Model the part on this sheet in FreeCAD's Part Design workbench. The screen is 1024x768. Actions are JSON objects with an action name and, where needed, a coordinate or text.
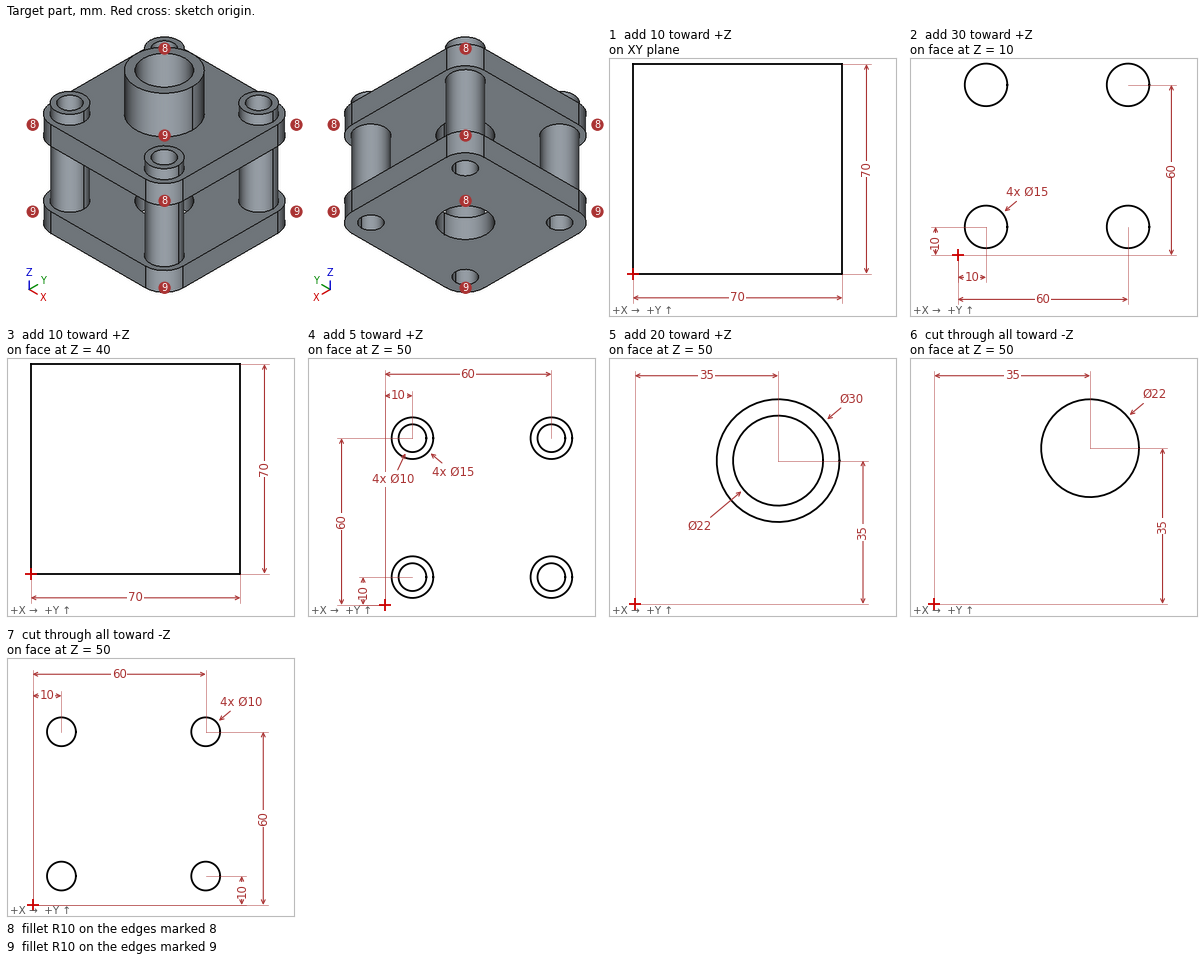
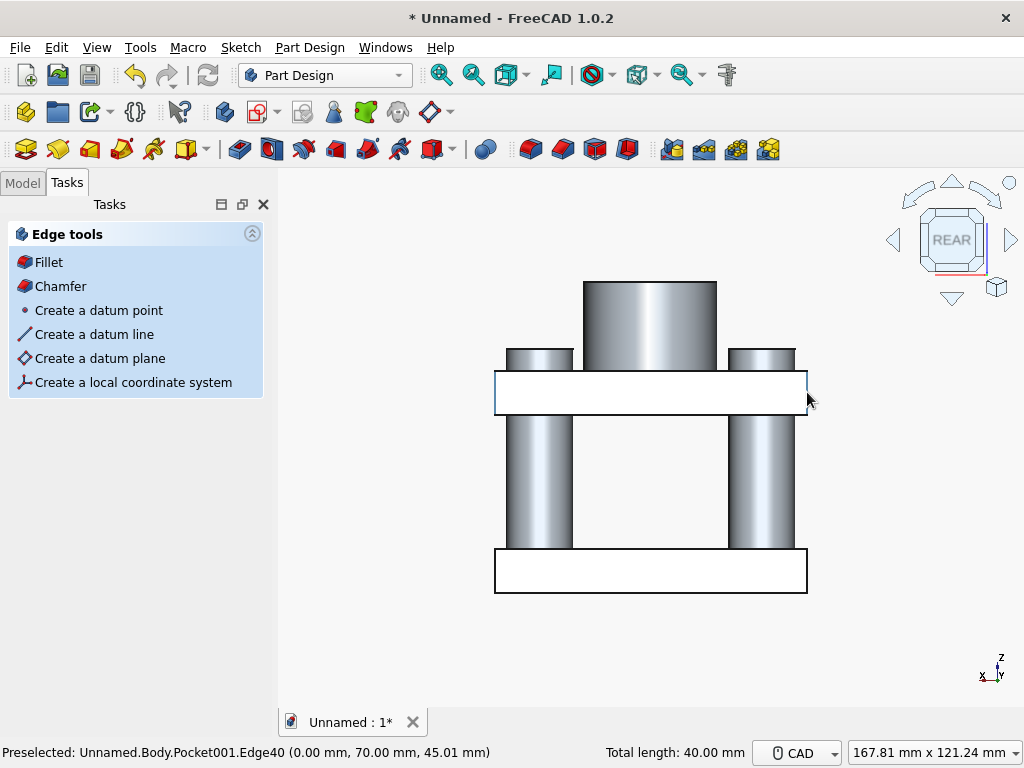
{"action": "left_click", "coordinate": [532, 150]}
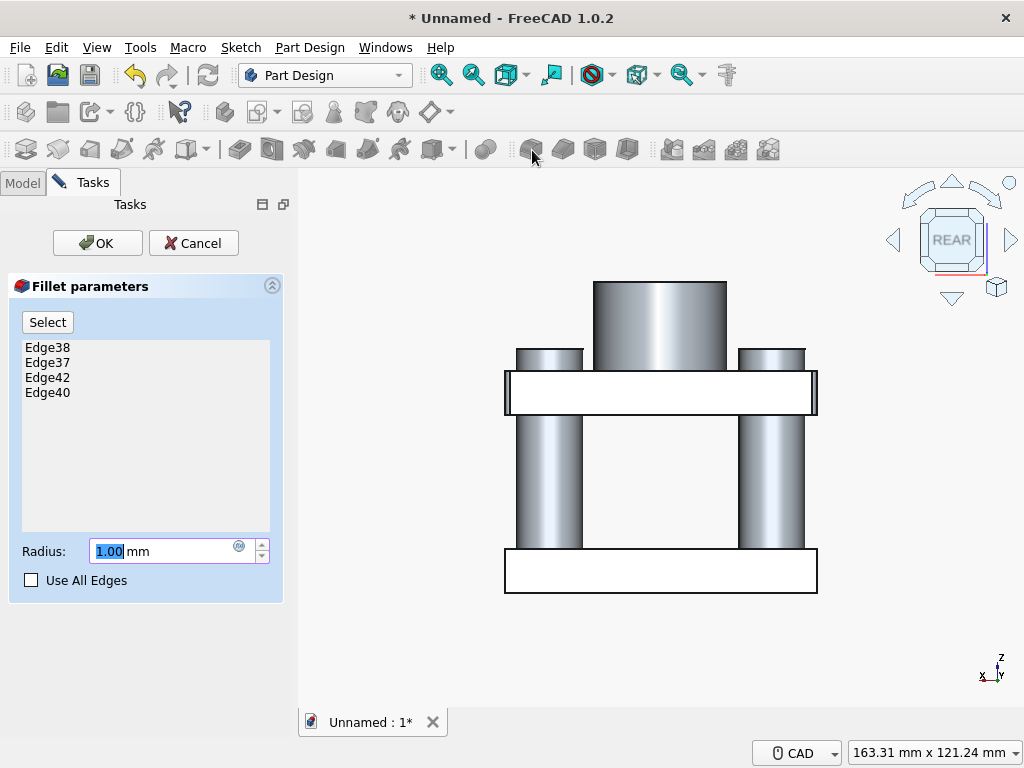
{"action": "type", "text": "10"}
{"action": "key", "text": "Tab"}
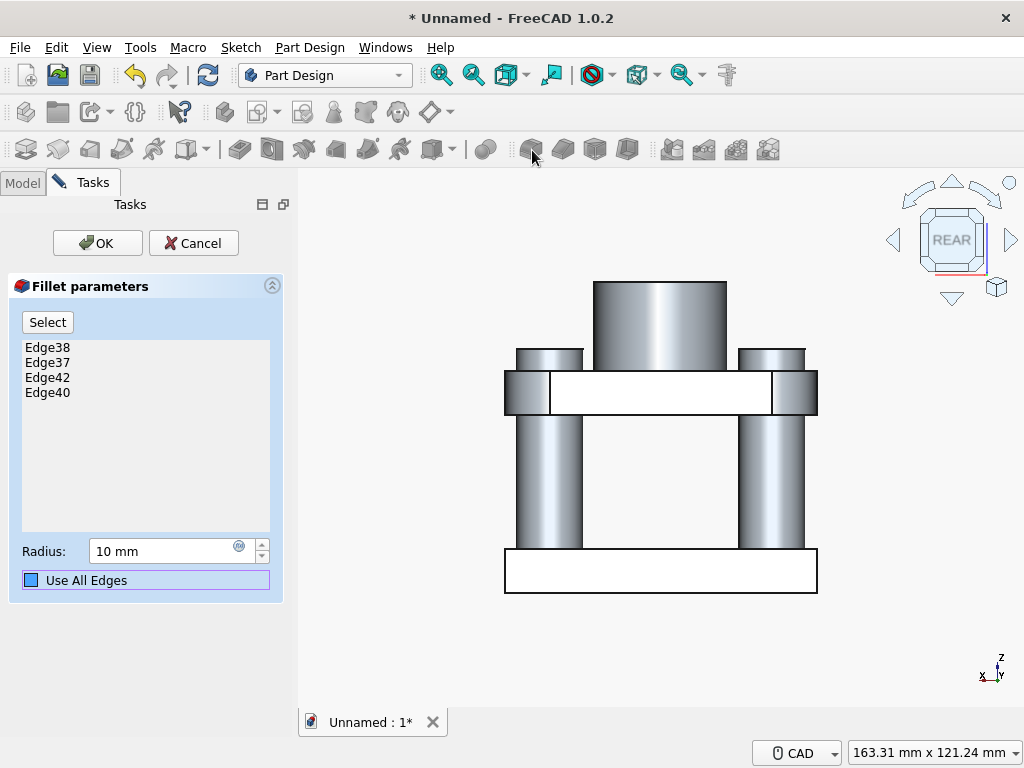
{"action": "left_click", "coordinate": [98, 243]}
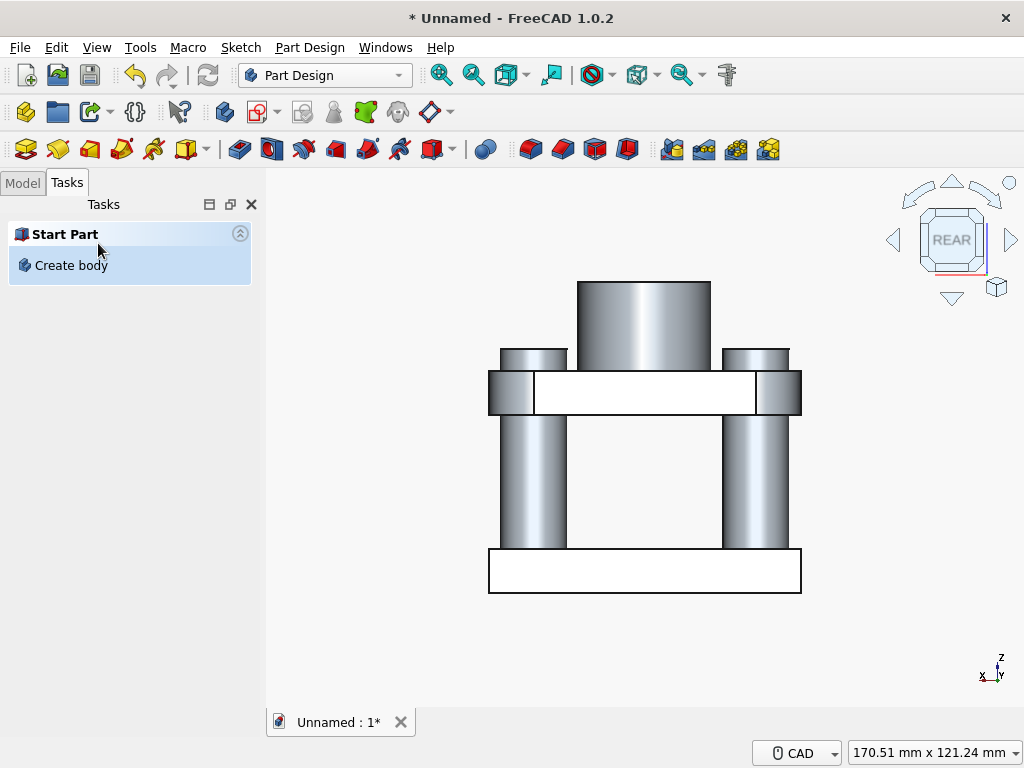
{"action": "left_click", "coordinate": [801, 570]}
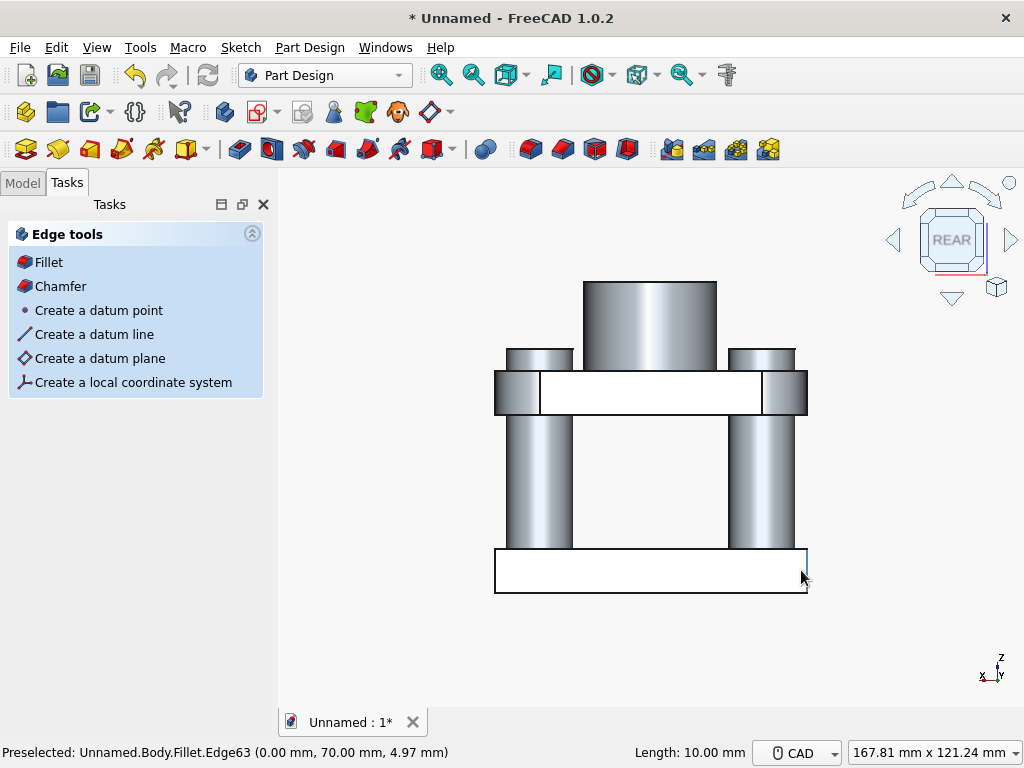
{"action": "left_click", "coordinate": [495, 570], "text": "ctrl"}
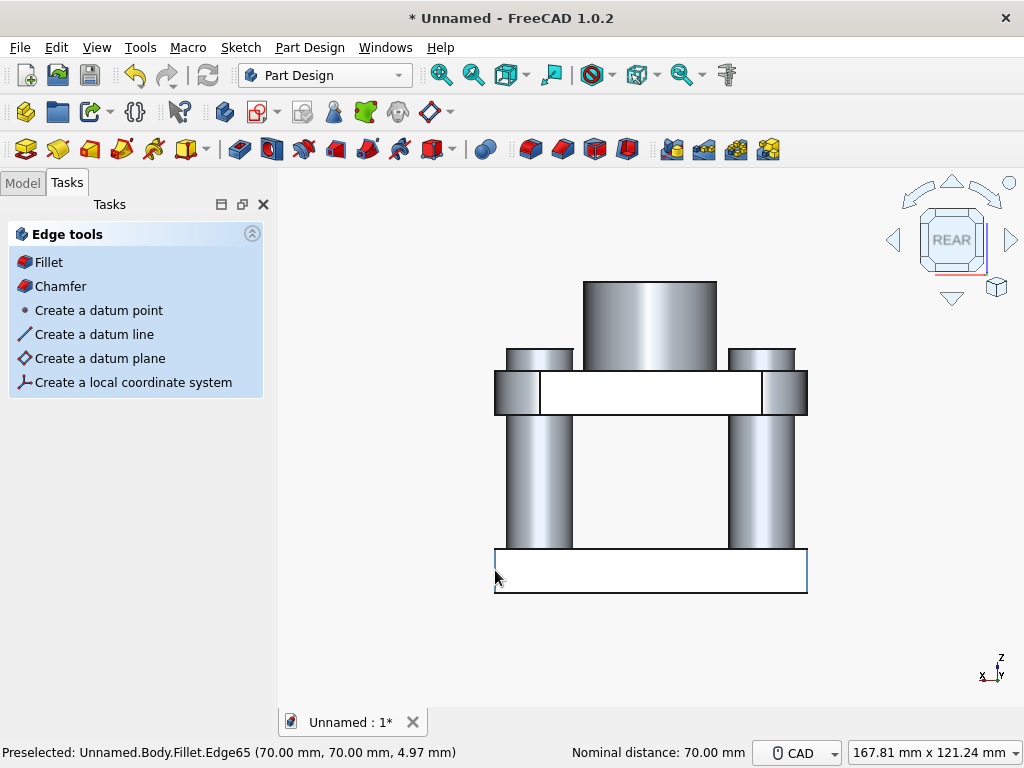
{"action": "key", "text": "0"}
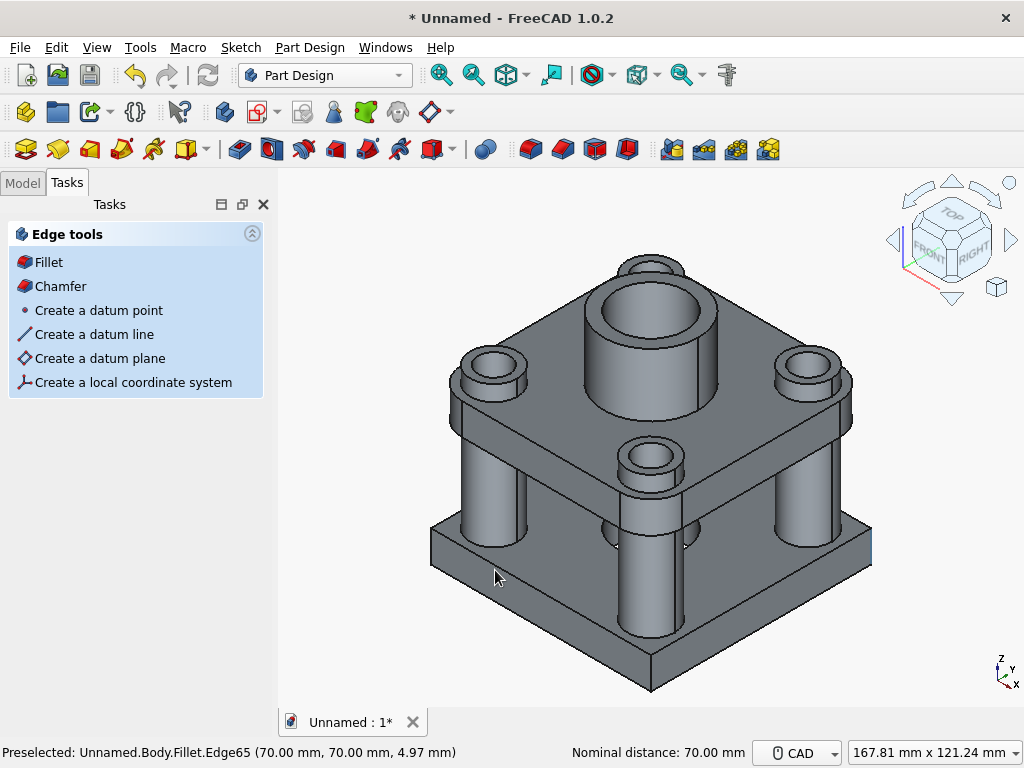
{"action": "left_click", "coordinate": [651, 672], "text": "ctrl"}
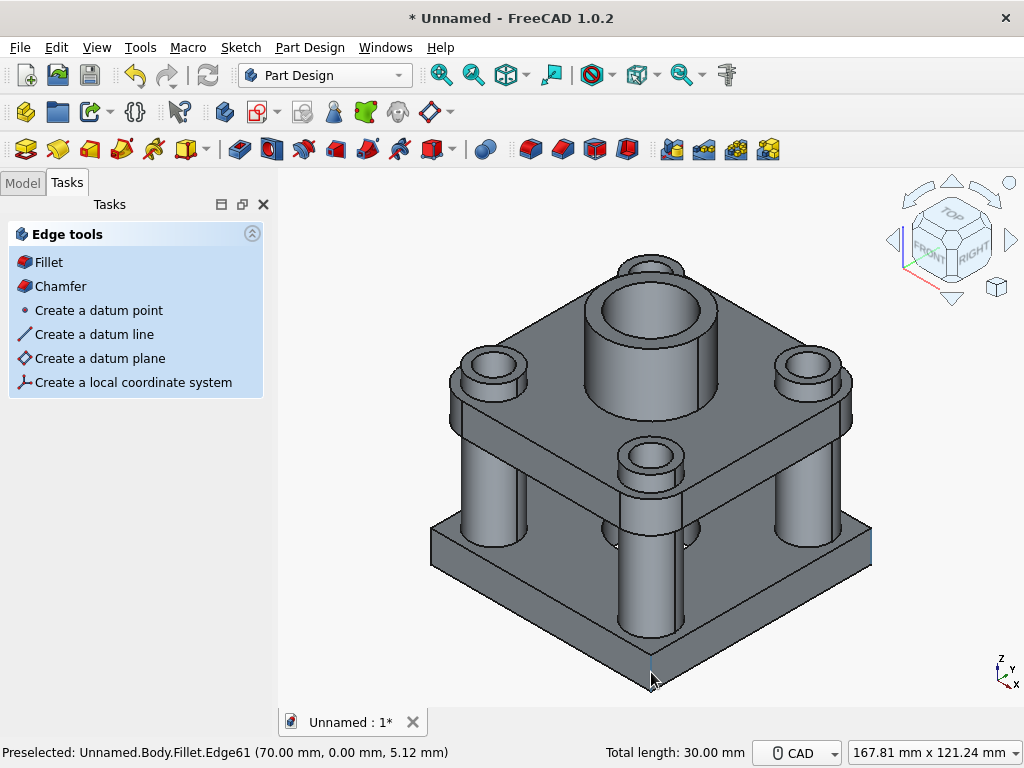
{"action": "key", "text": "2"}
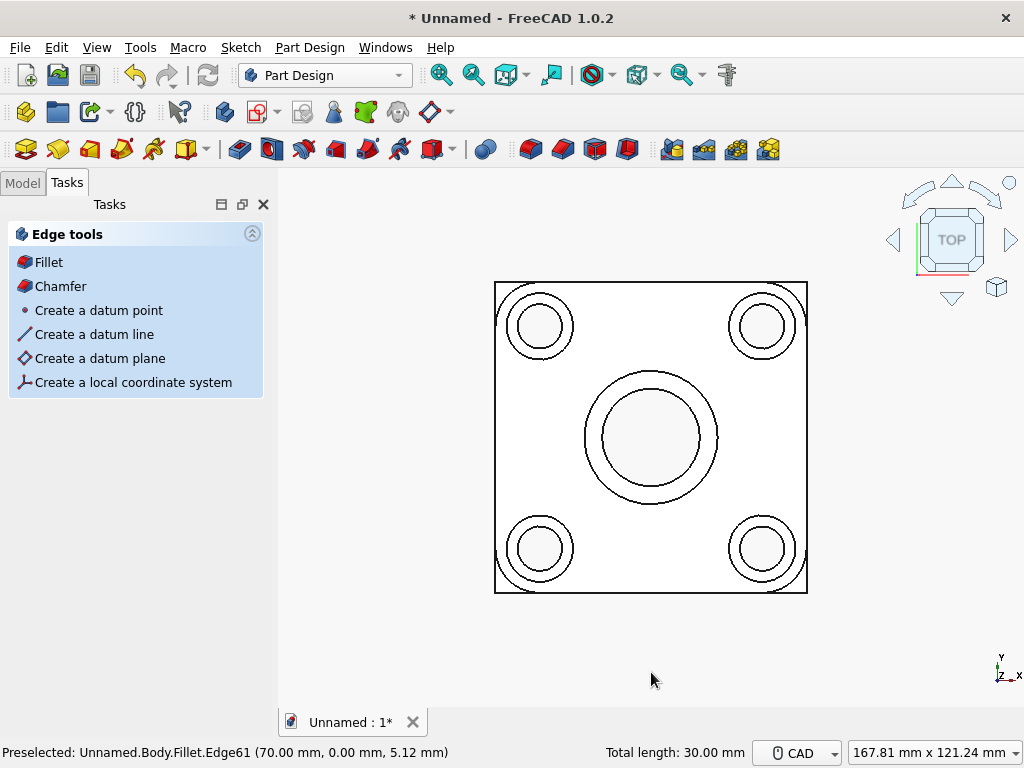
{"action": "key", "text": "1"}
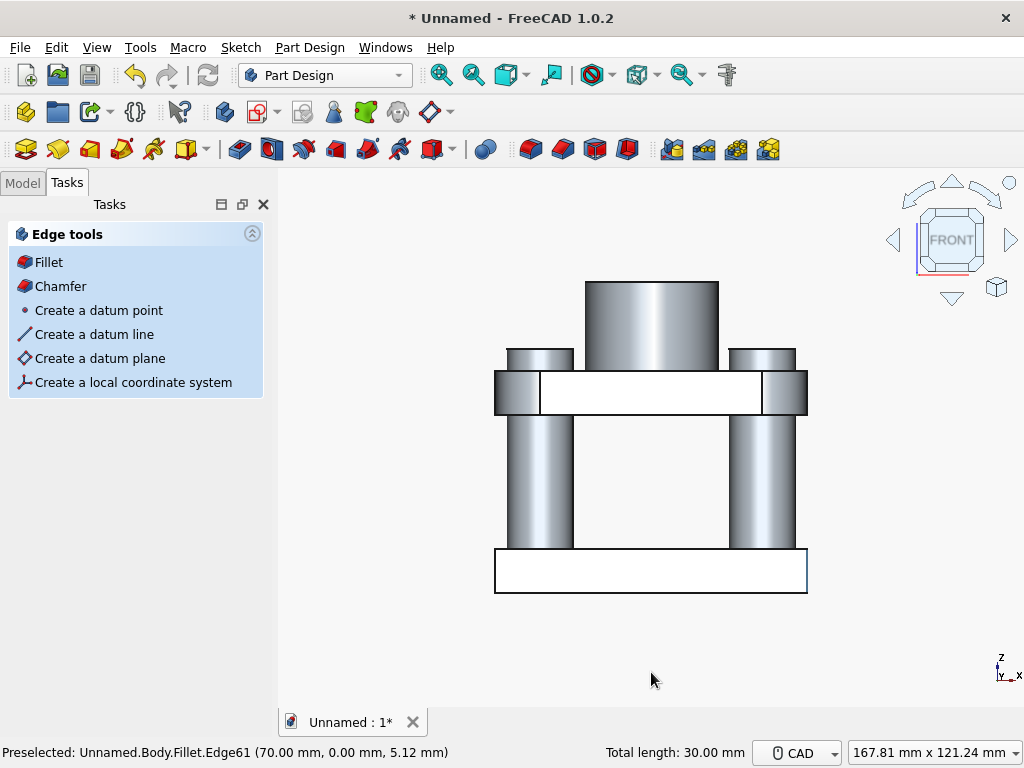
{"action": "left_click", "coordinate": [495, 570], "text": "ctrl"}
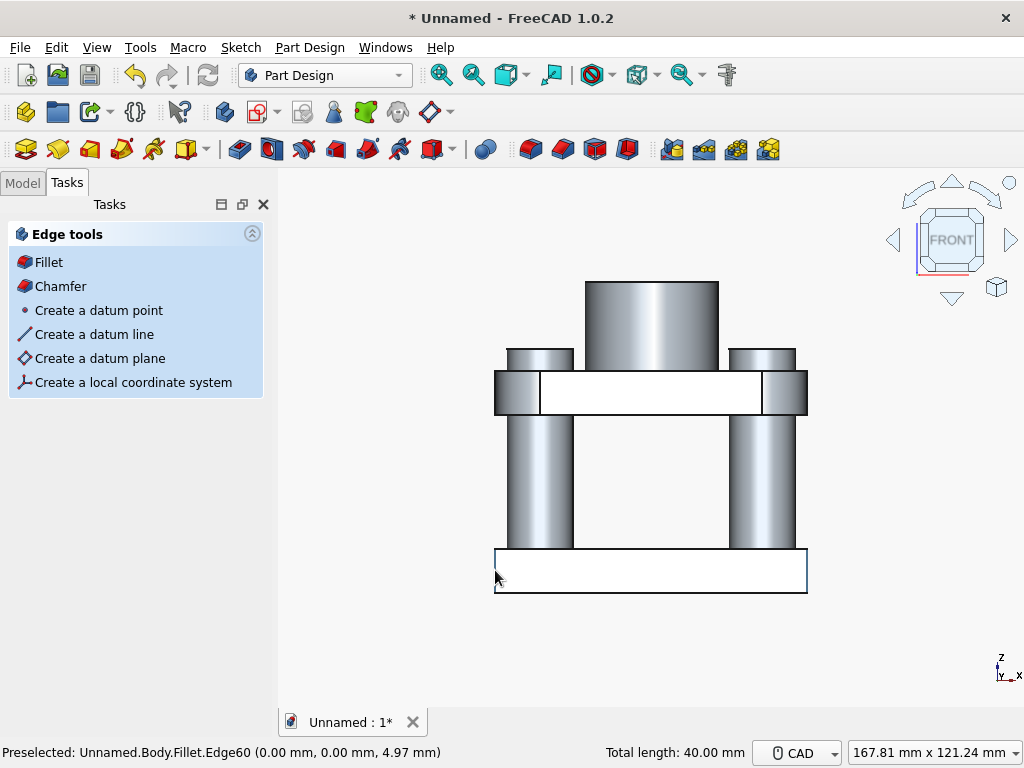
{"action": "left_click", "coordinate": [532, 150]}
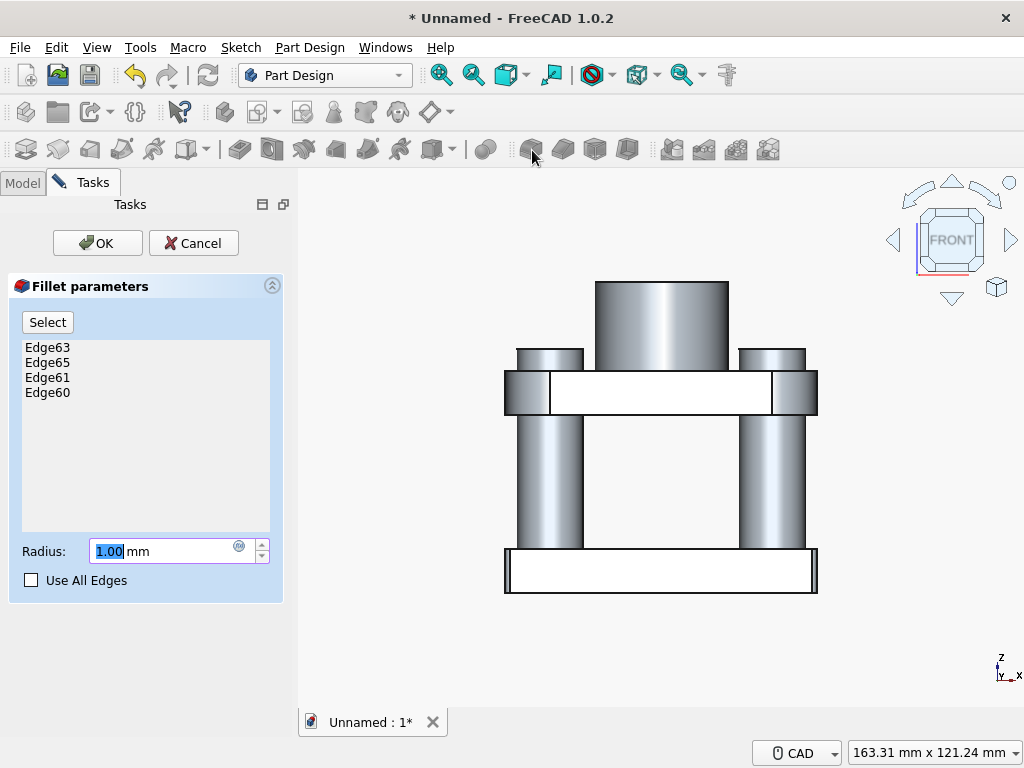
{"action": "type", "text": "10"}
{"action": "key", "text": "Tab"}